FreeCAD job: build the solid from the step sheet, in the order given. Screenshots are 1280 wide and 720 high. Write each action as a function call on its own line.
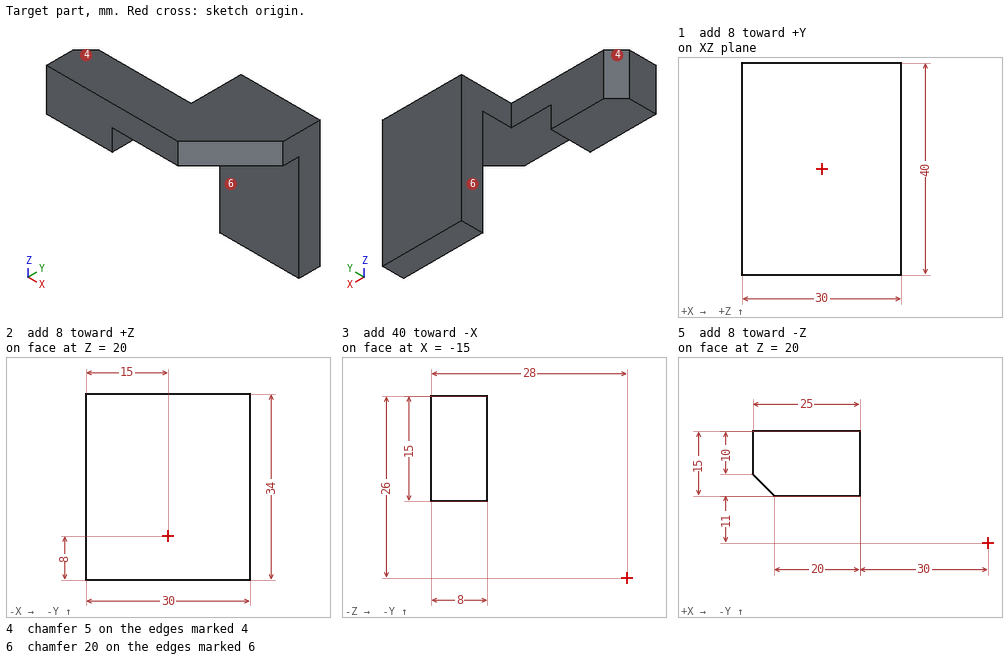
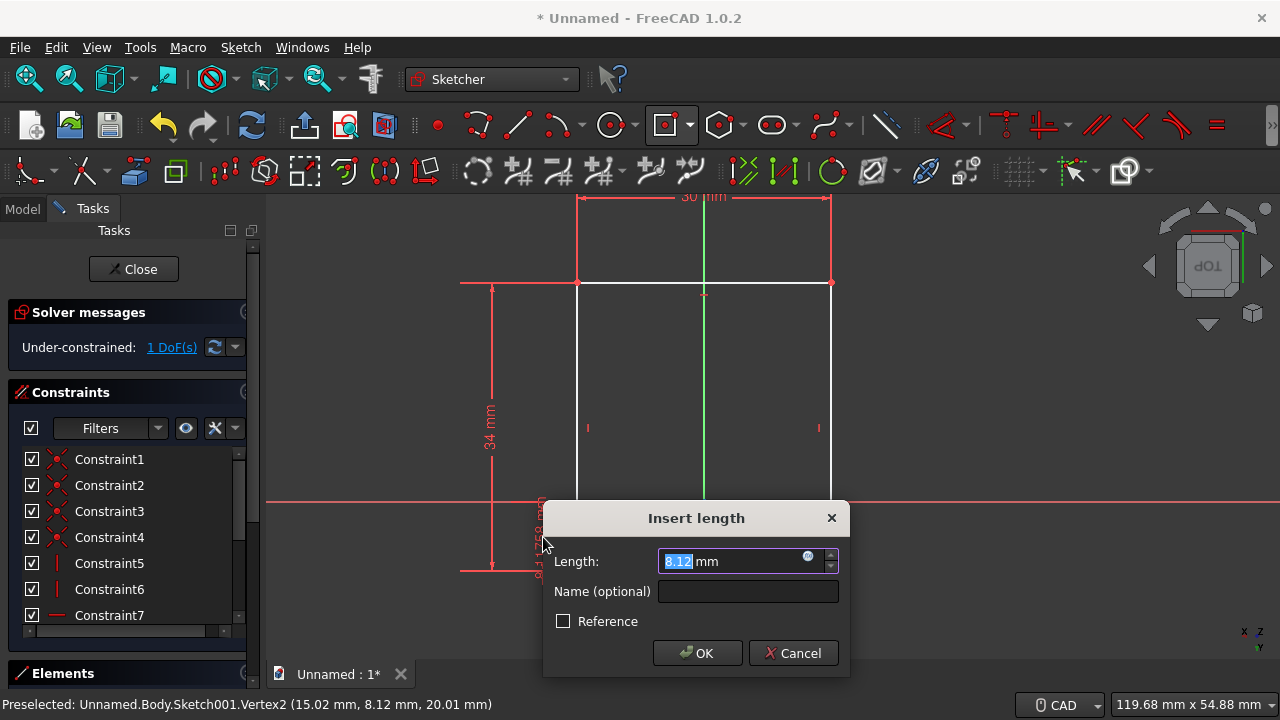
text(8)
key(Return)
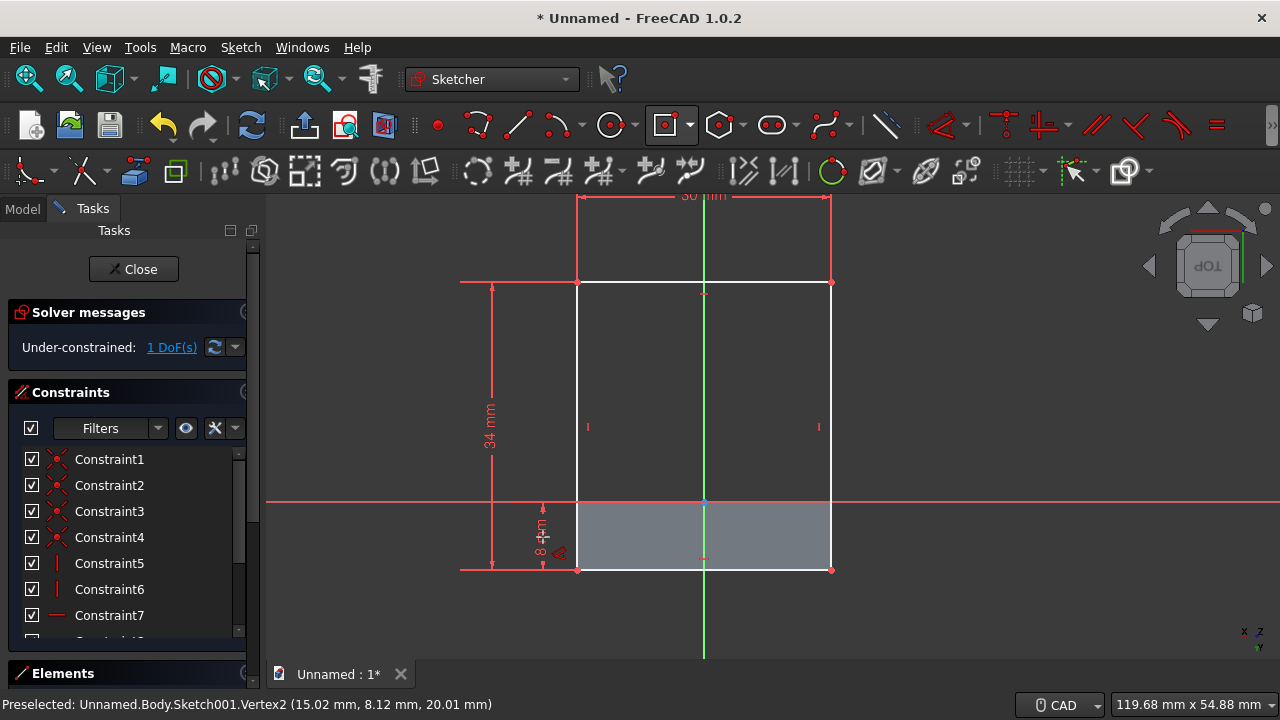
click(577, 282)
click(641, 248)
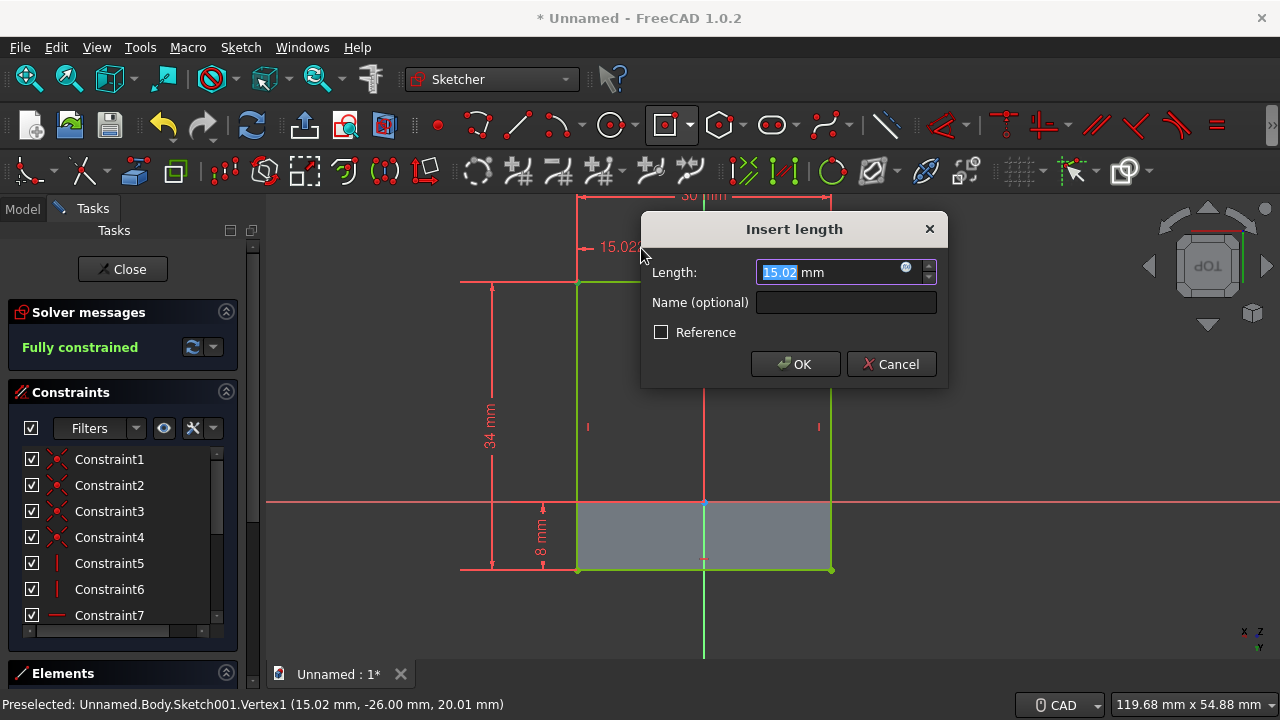
text(15)
key(Return)
key(Escape)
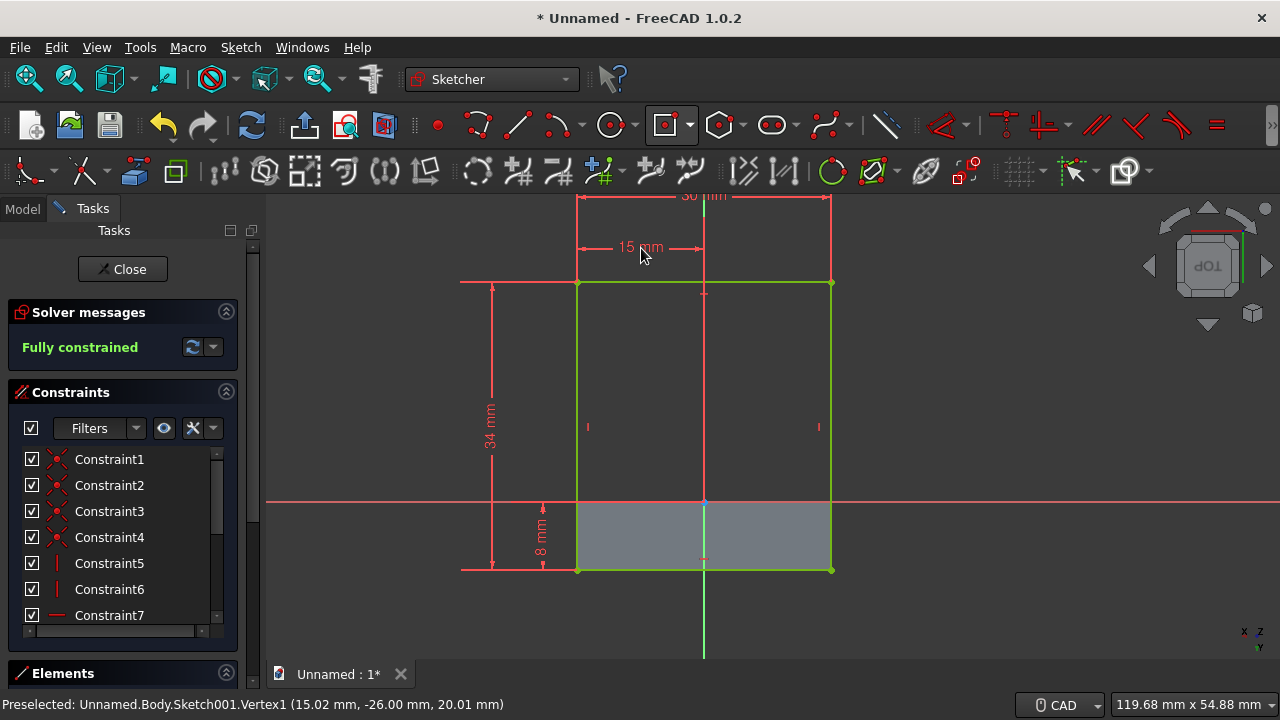
click(123, 269)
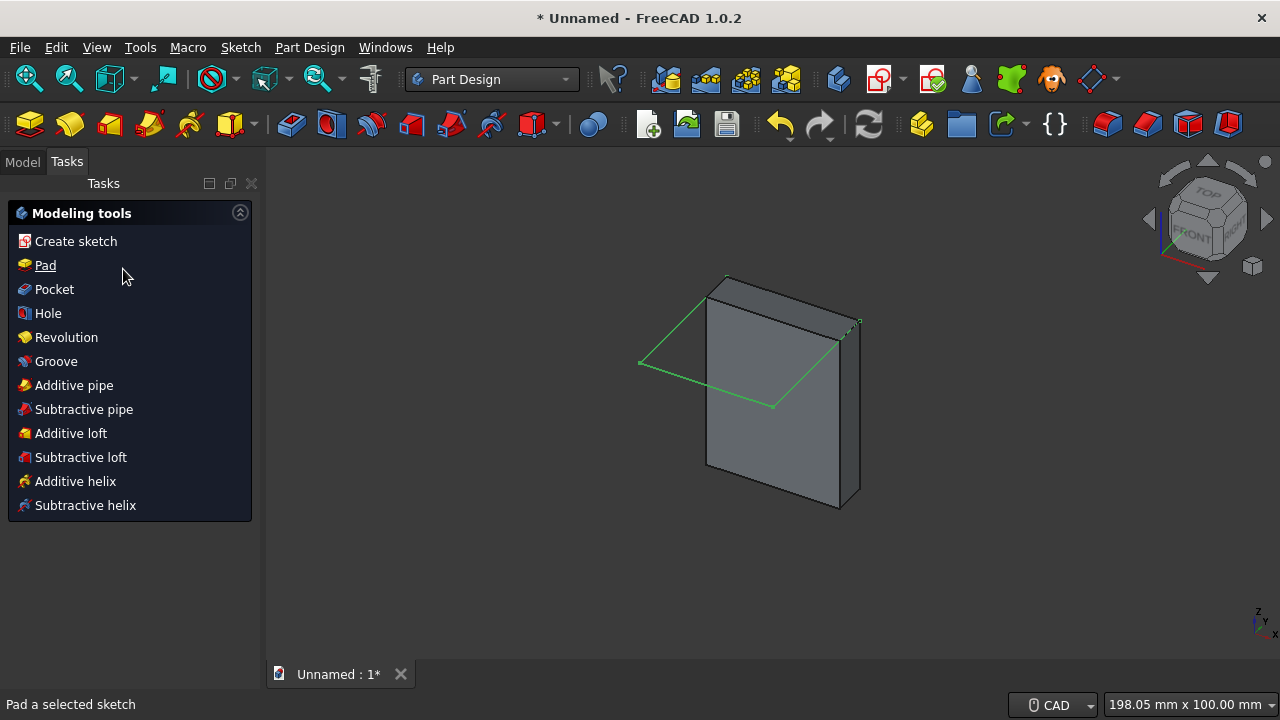
click(30, 124)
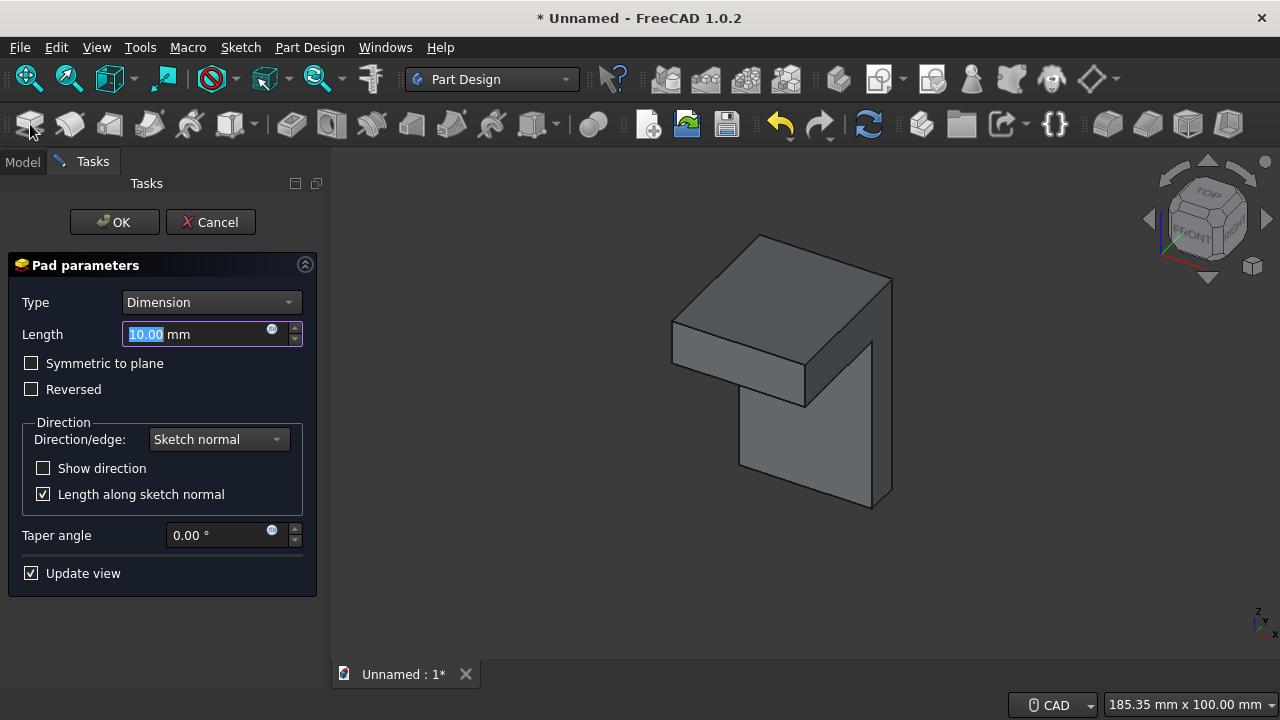
text(8)
key(Tab)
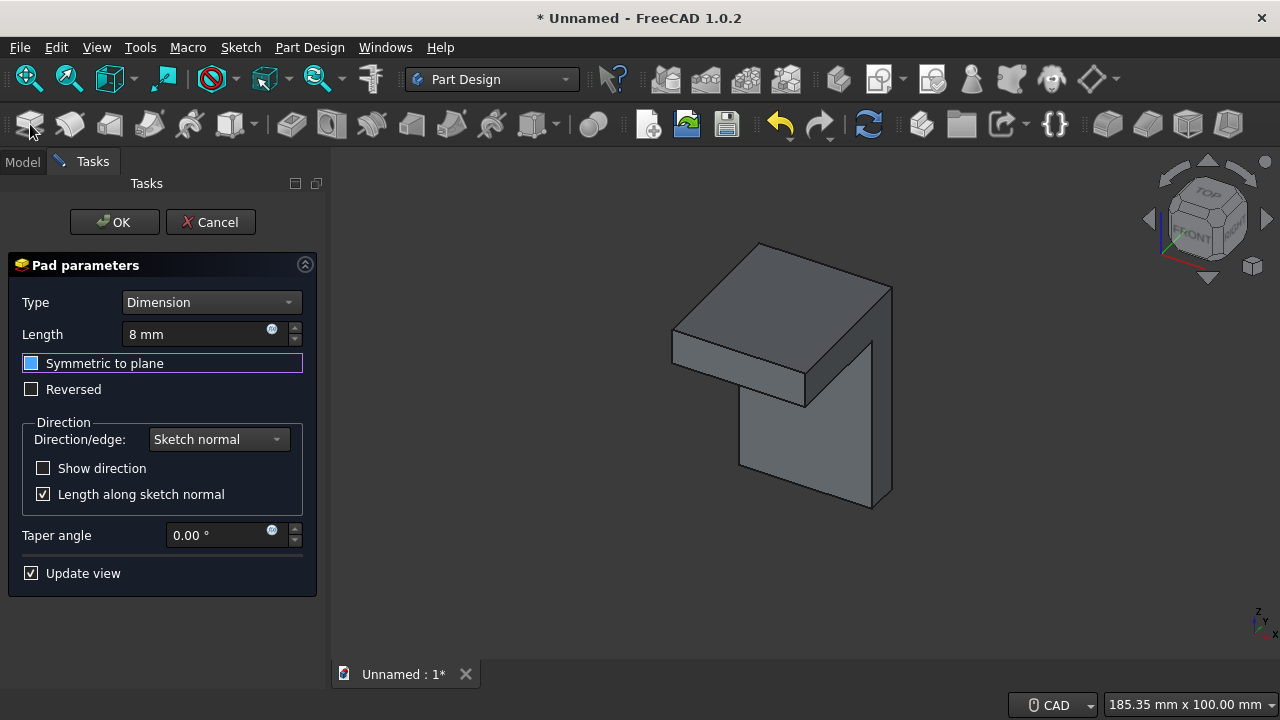
click(115, 222)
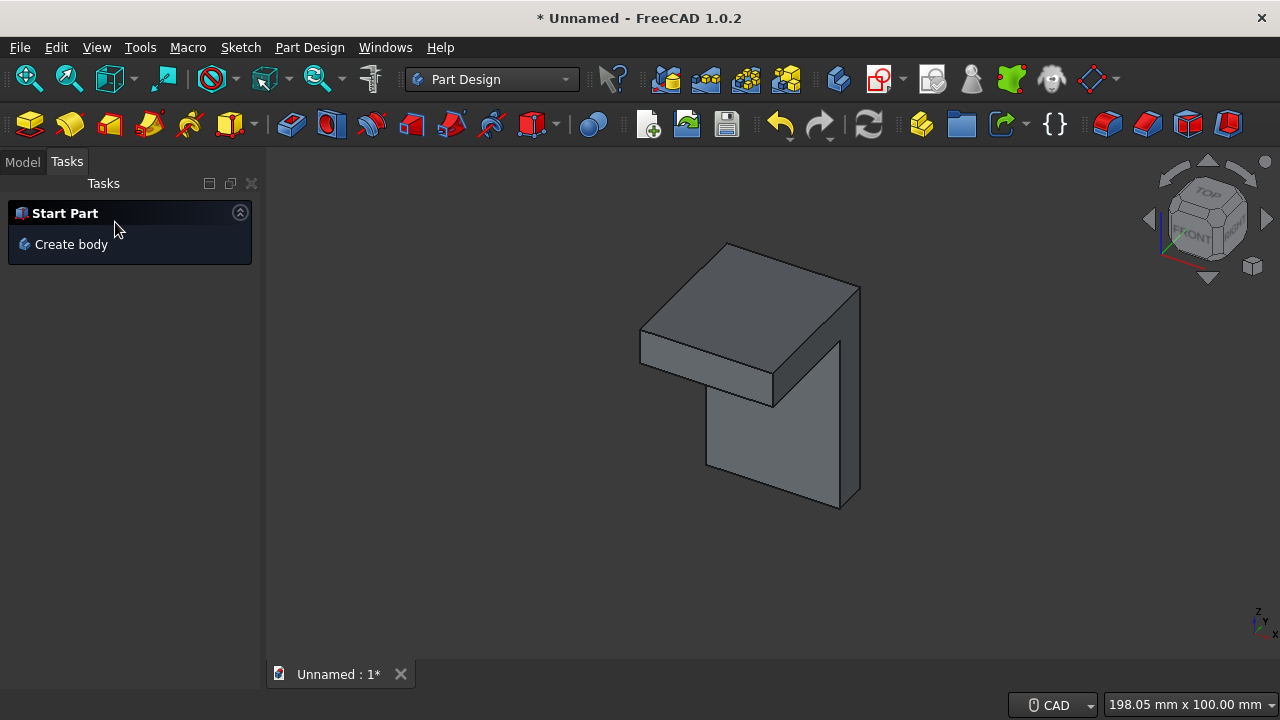
key(6)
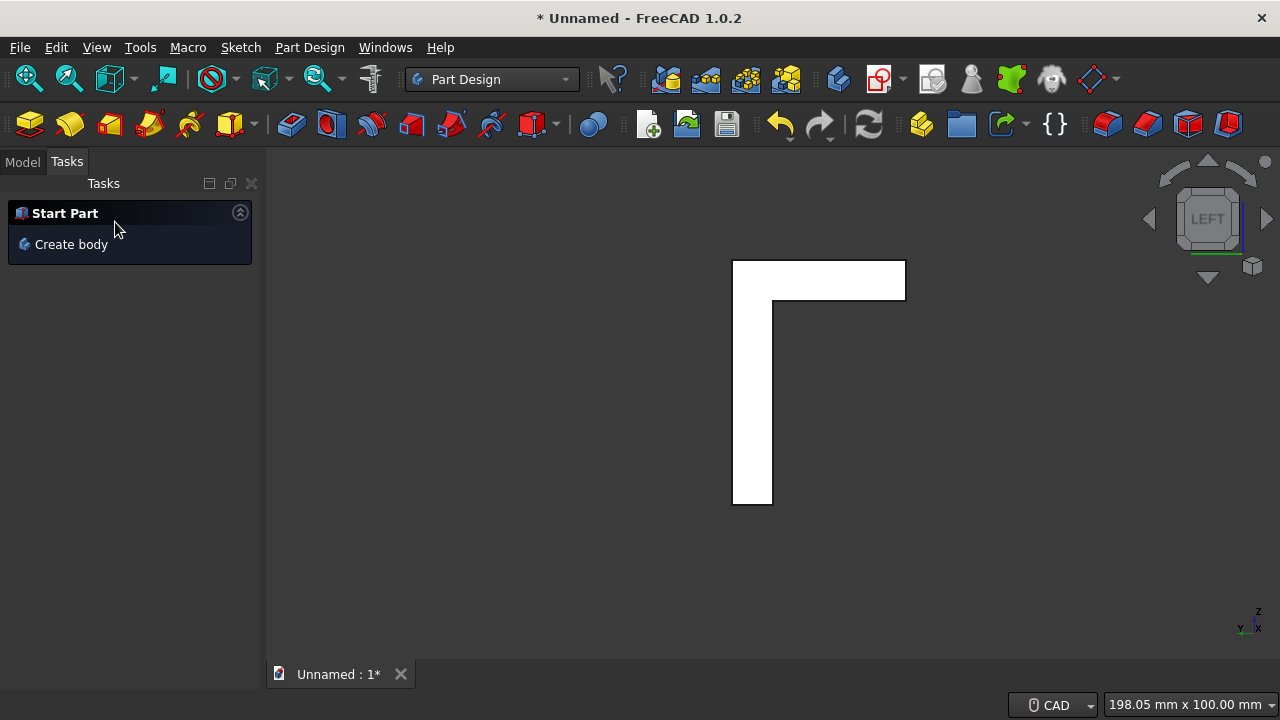
click(819, 276)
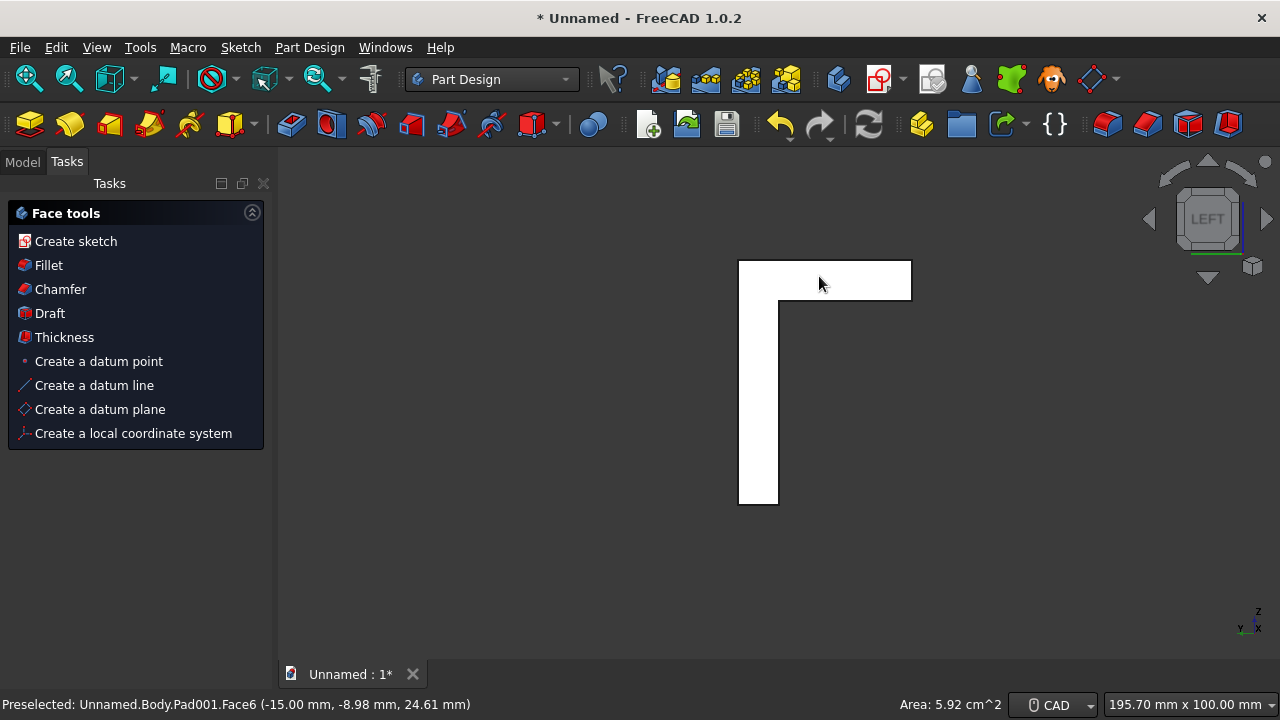
click(880, 80)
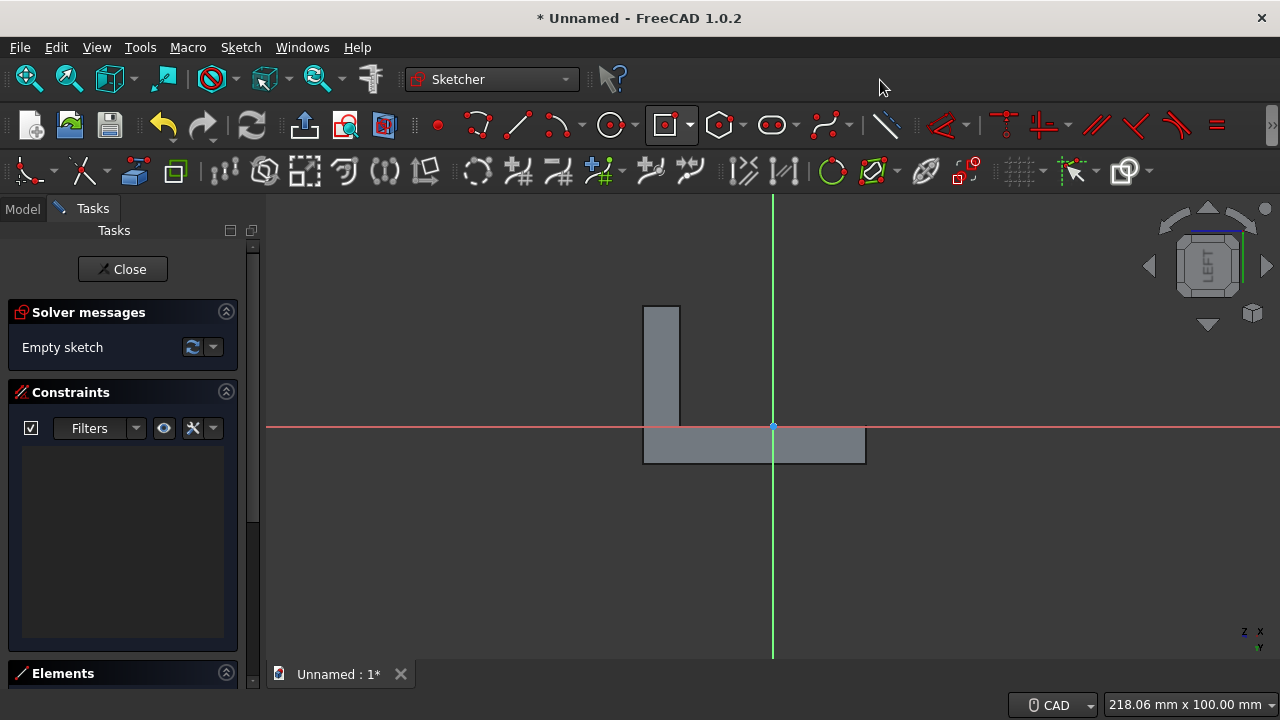
scroll(711, 317, up, 4)